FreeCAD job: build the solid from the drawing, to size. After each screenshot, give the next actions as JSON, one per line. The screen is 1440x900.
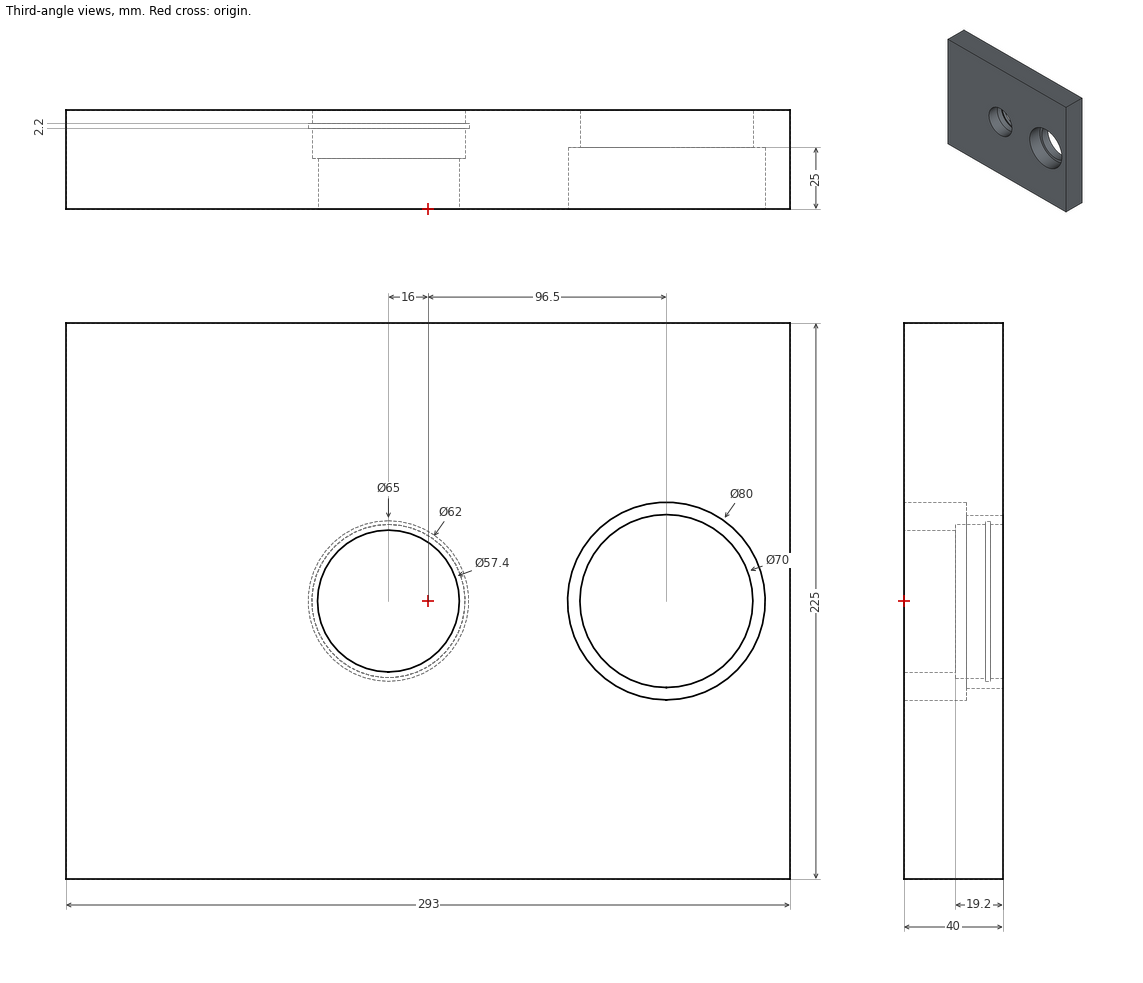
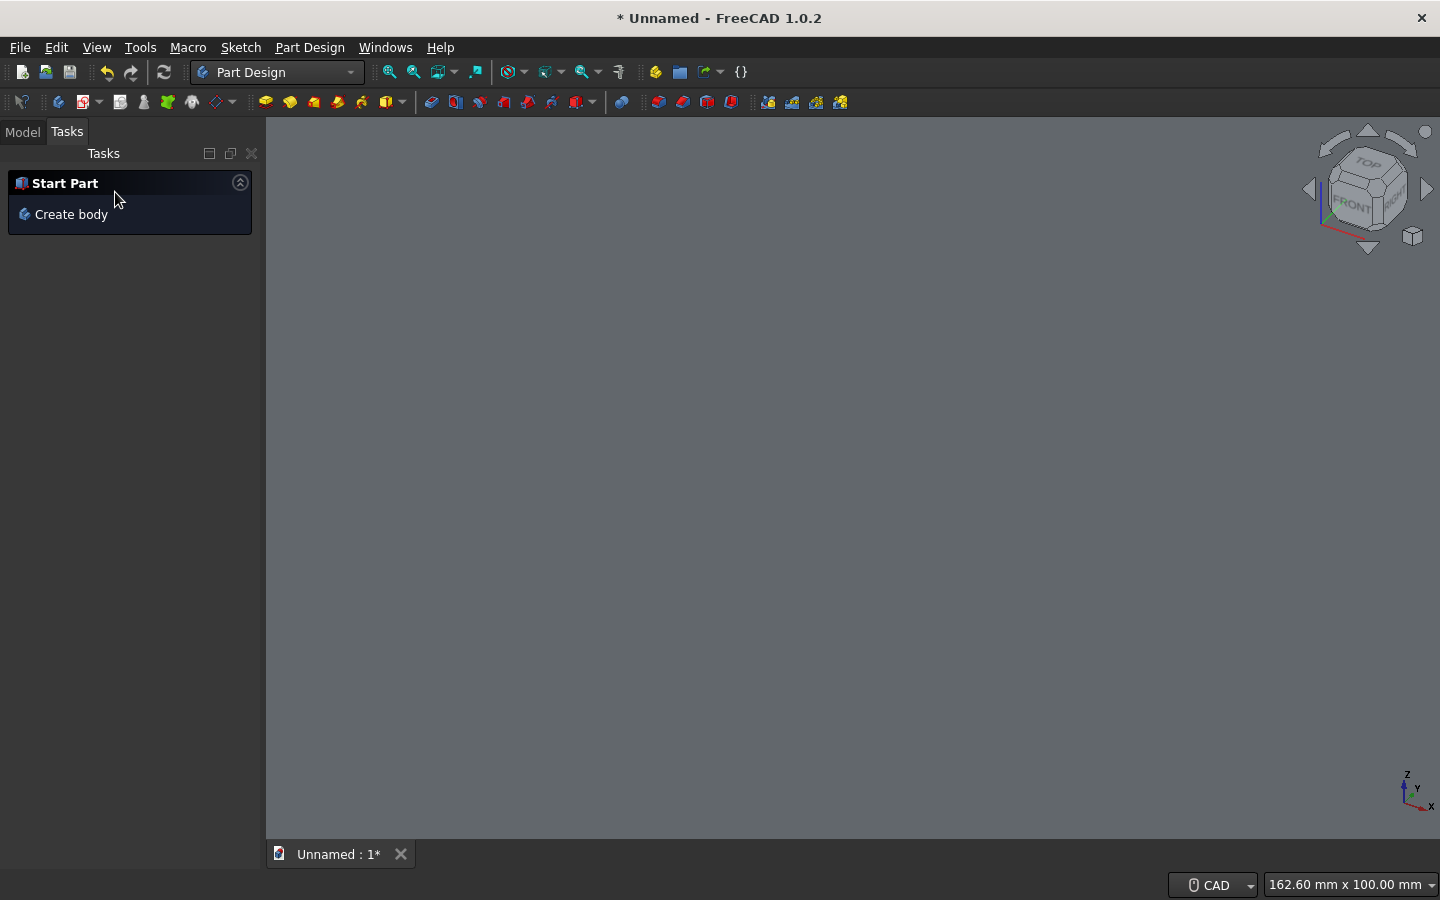
{"action": "left_click", "coordinate": [390, 72]}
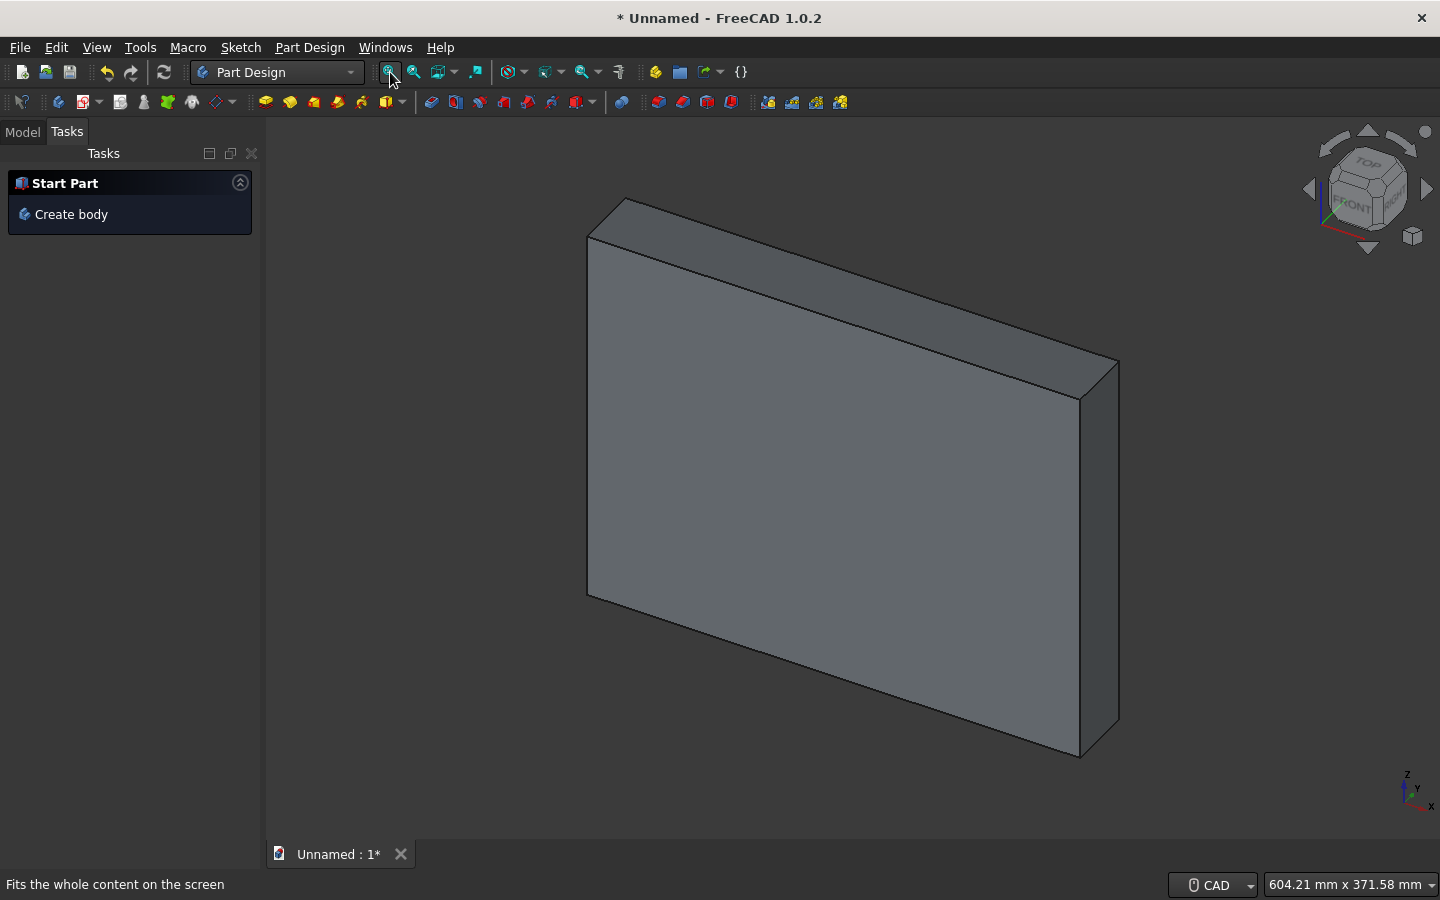
{"action": "left_click", "coordinate": [84, 102]}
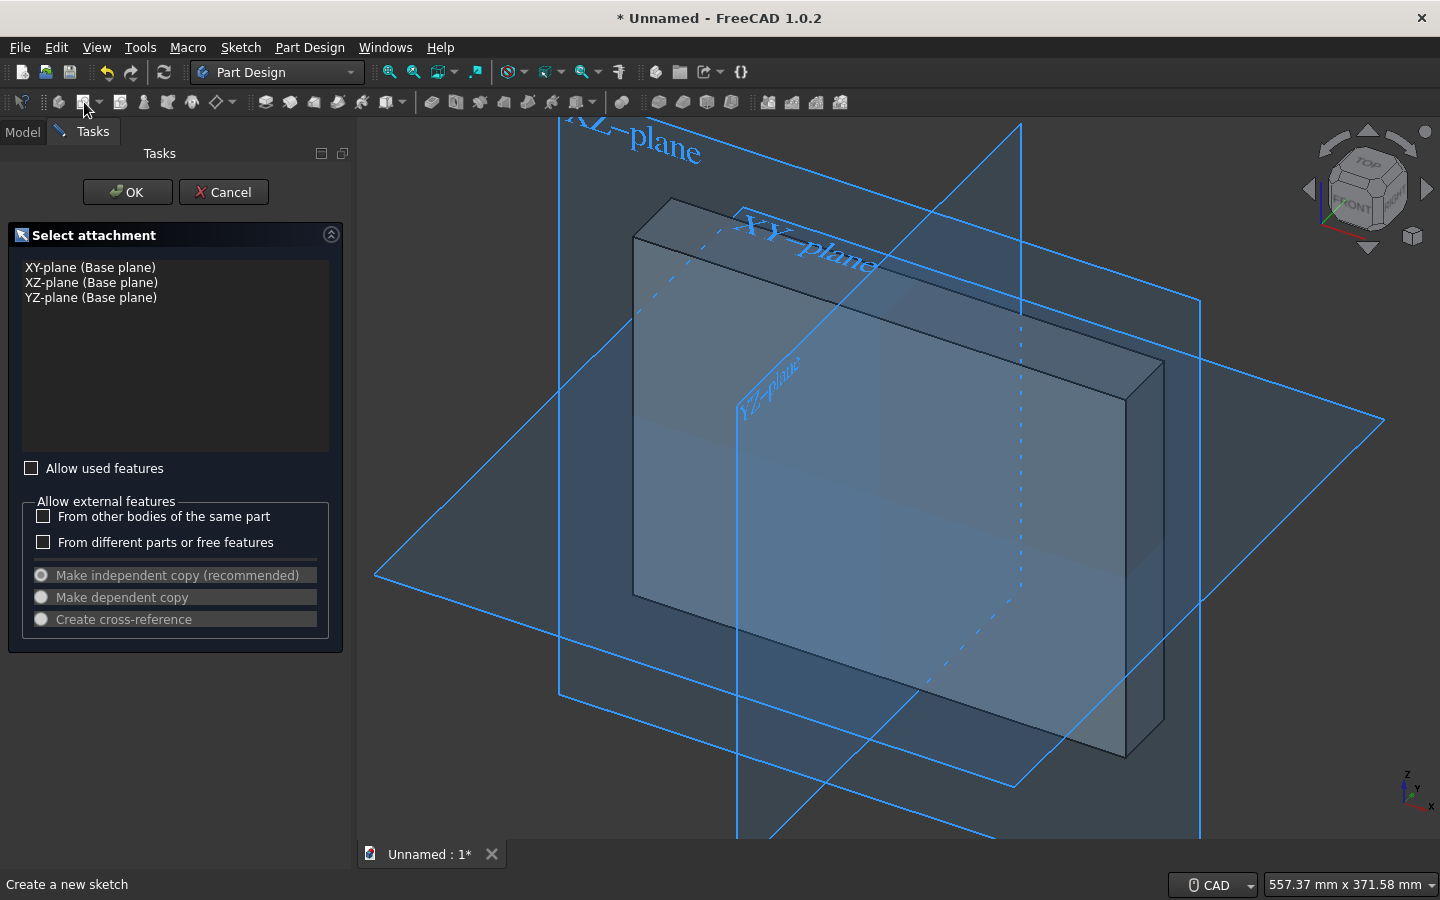
{"action": "left_click", "coordinate": [82, 282]}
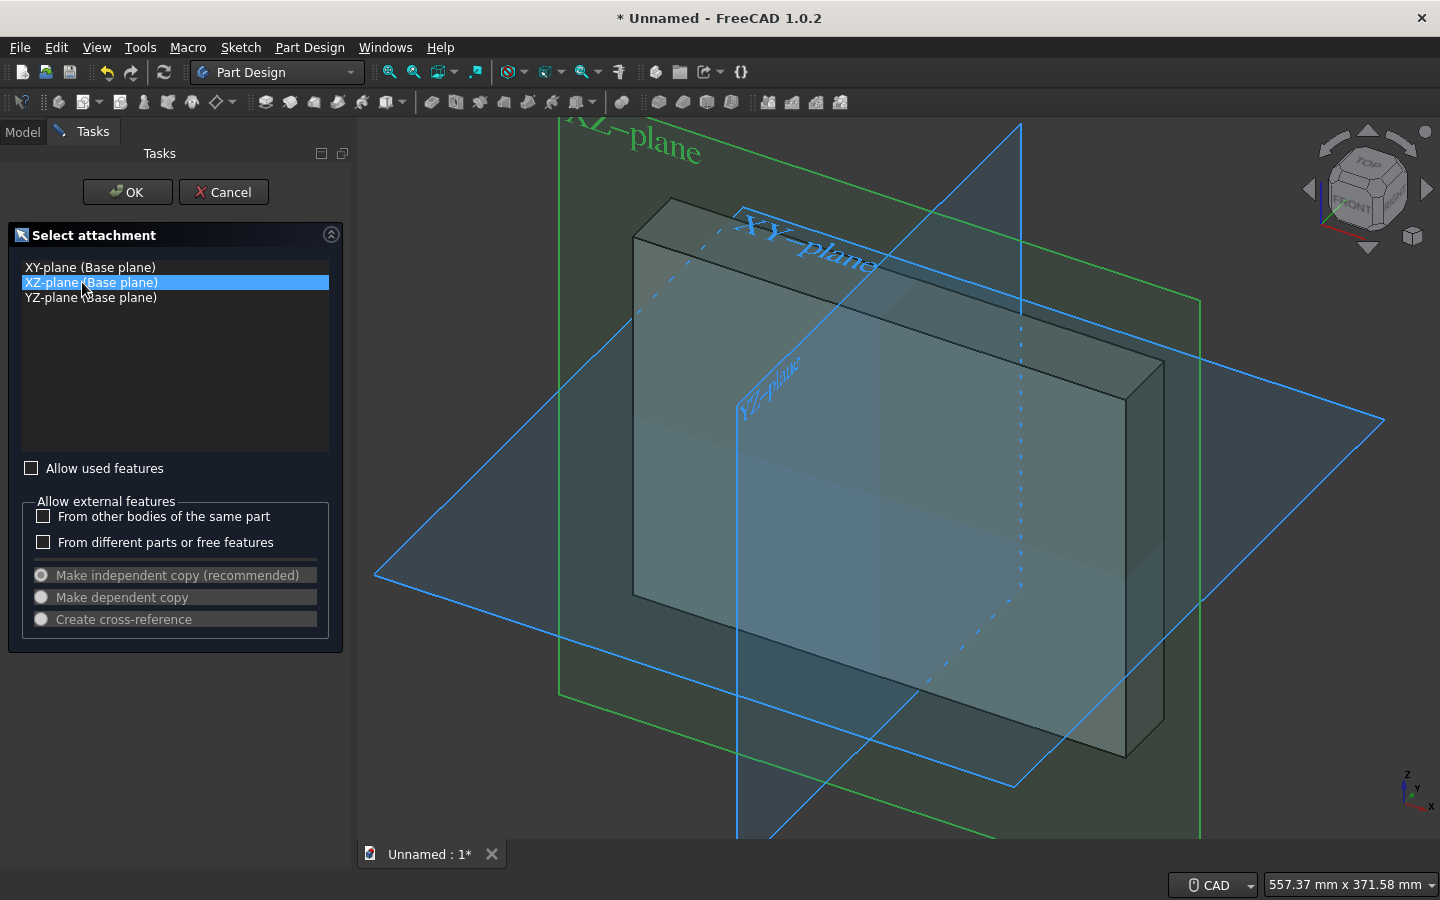
{"action": "left_click", "coordinate": [128, 192]}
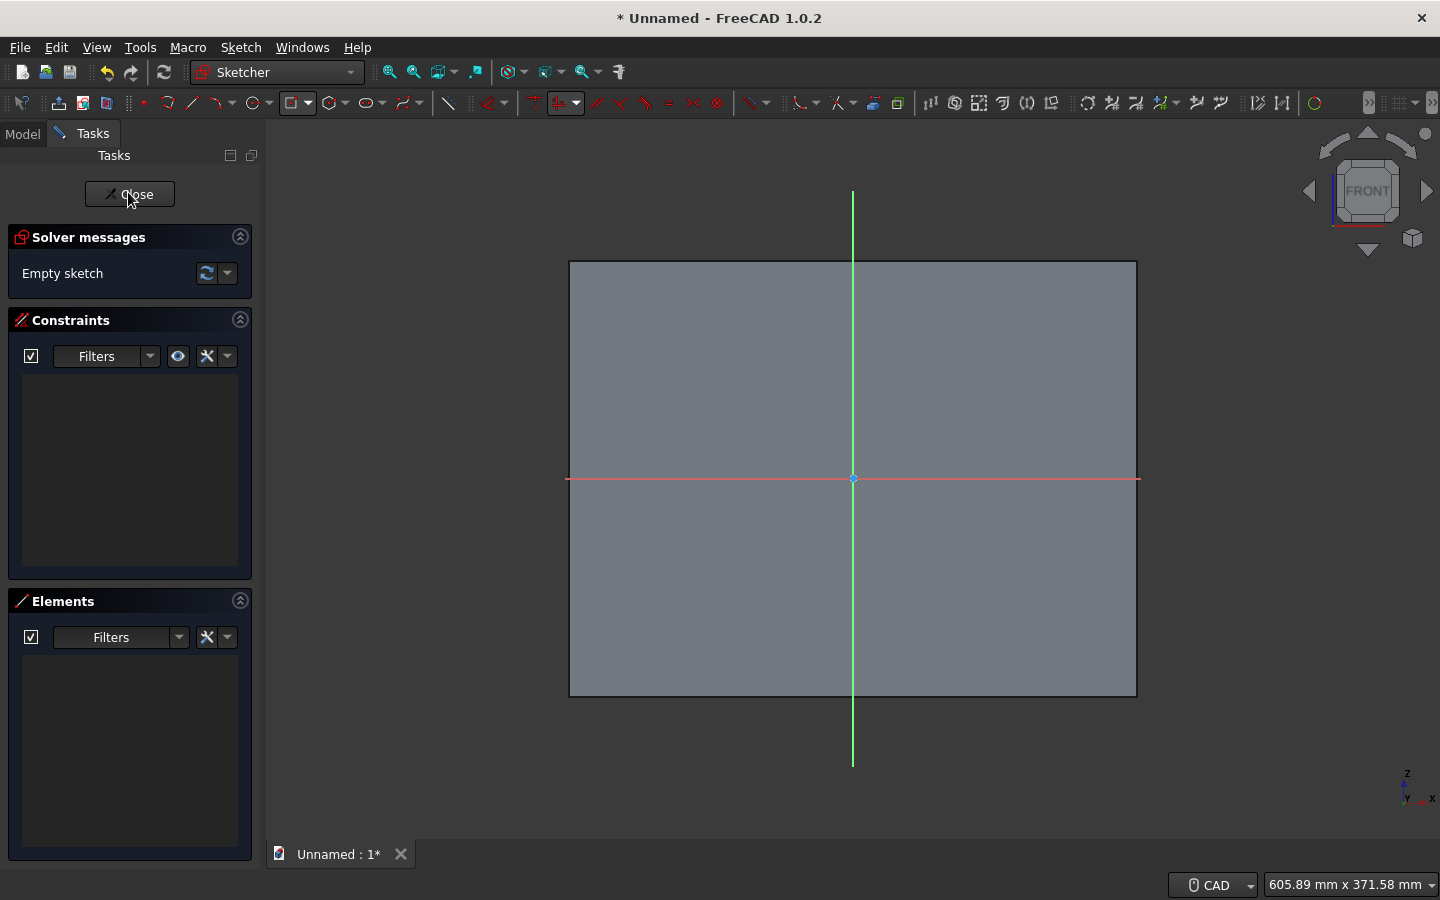
{"action": "scroll", "coordinate": [1102, 479], "scroll_direction": "up", "scroll_amount": 5}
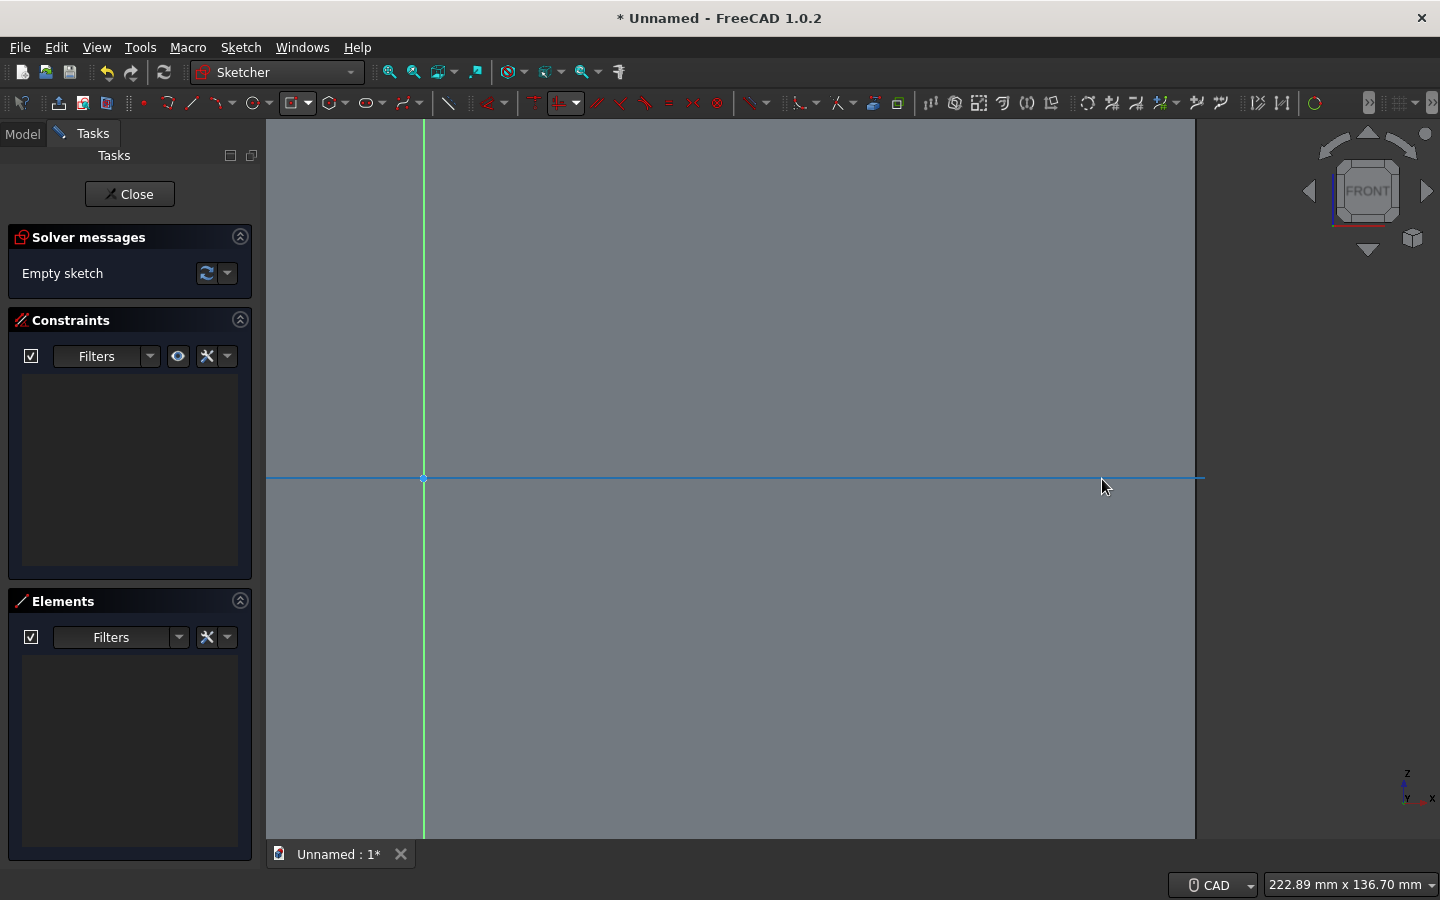
{"action": "left_click", "coordinate": [254, 104]}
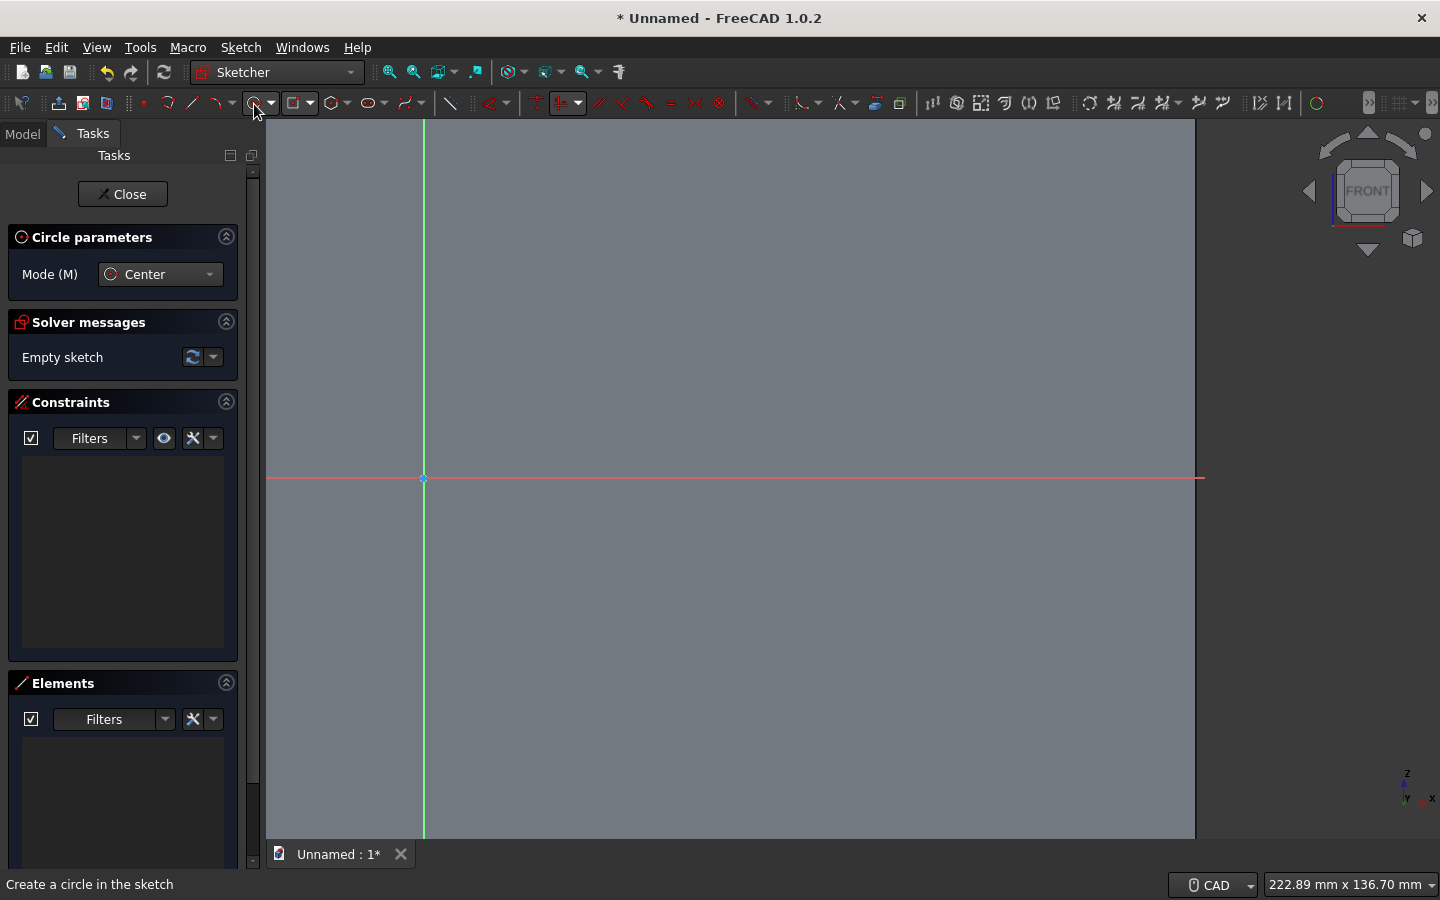
{"action": "left_click", "coordinate": [932, 478]}
{"action": "mouse_move", "coordinate": [1081, 329]}